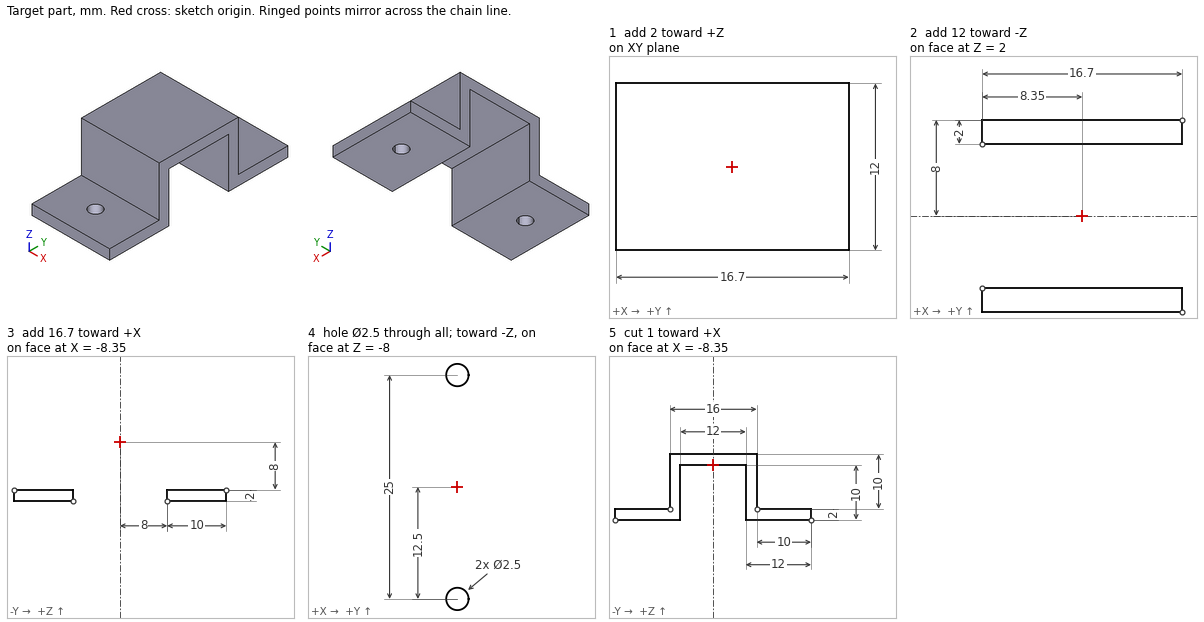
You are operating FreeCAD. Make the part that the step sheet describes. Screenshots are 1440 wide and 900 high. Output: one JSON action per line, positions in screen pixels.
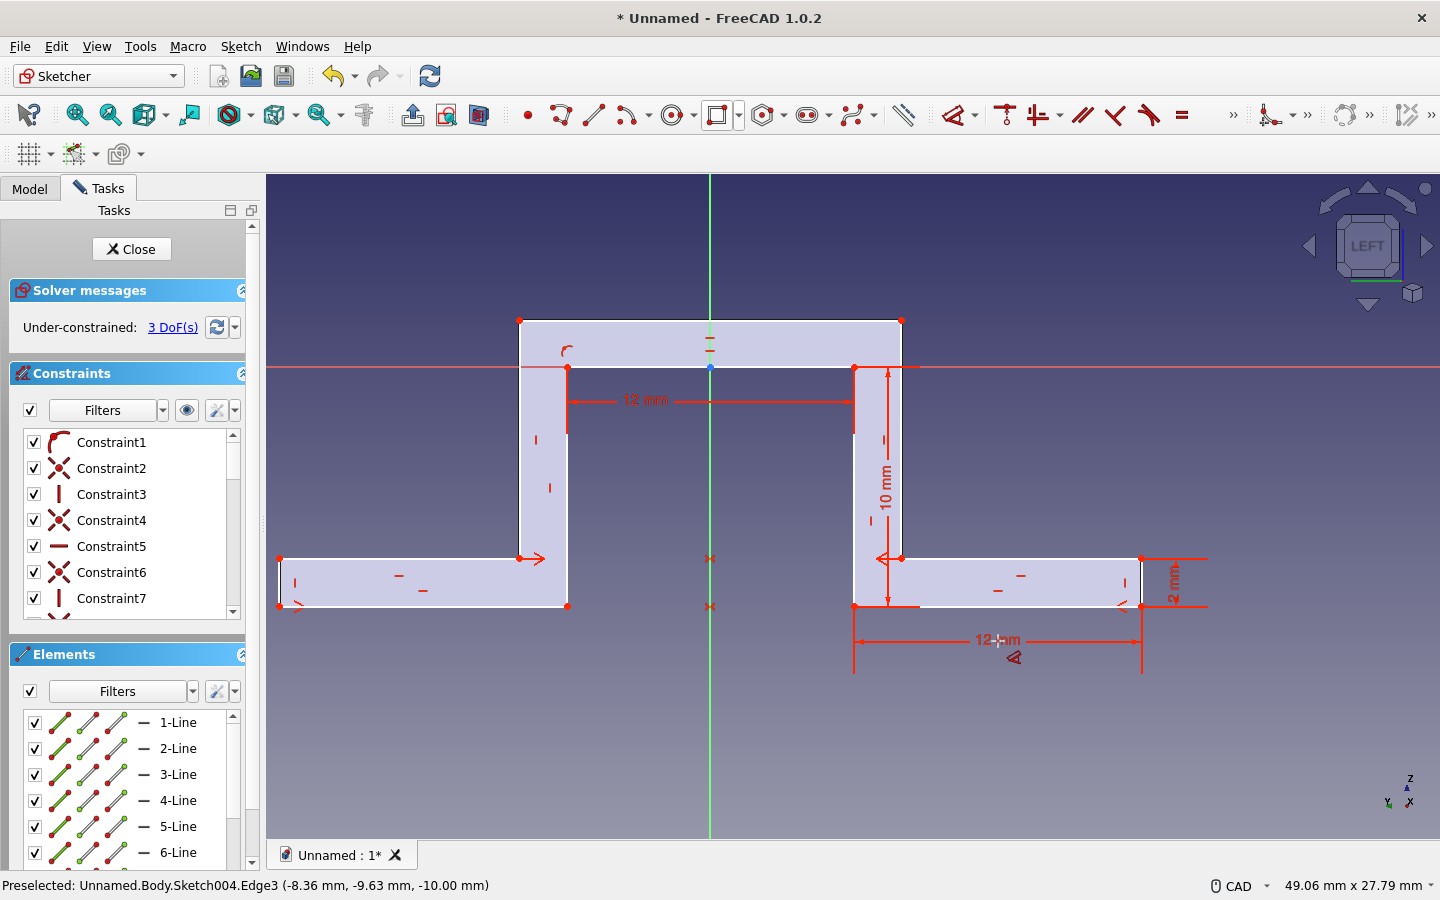
{"action": "left_click", "coordinate": [1070, 559]}
{"action": "left_click", "coordinate": [1022, 593]}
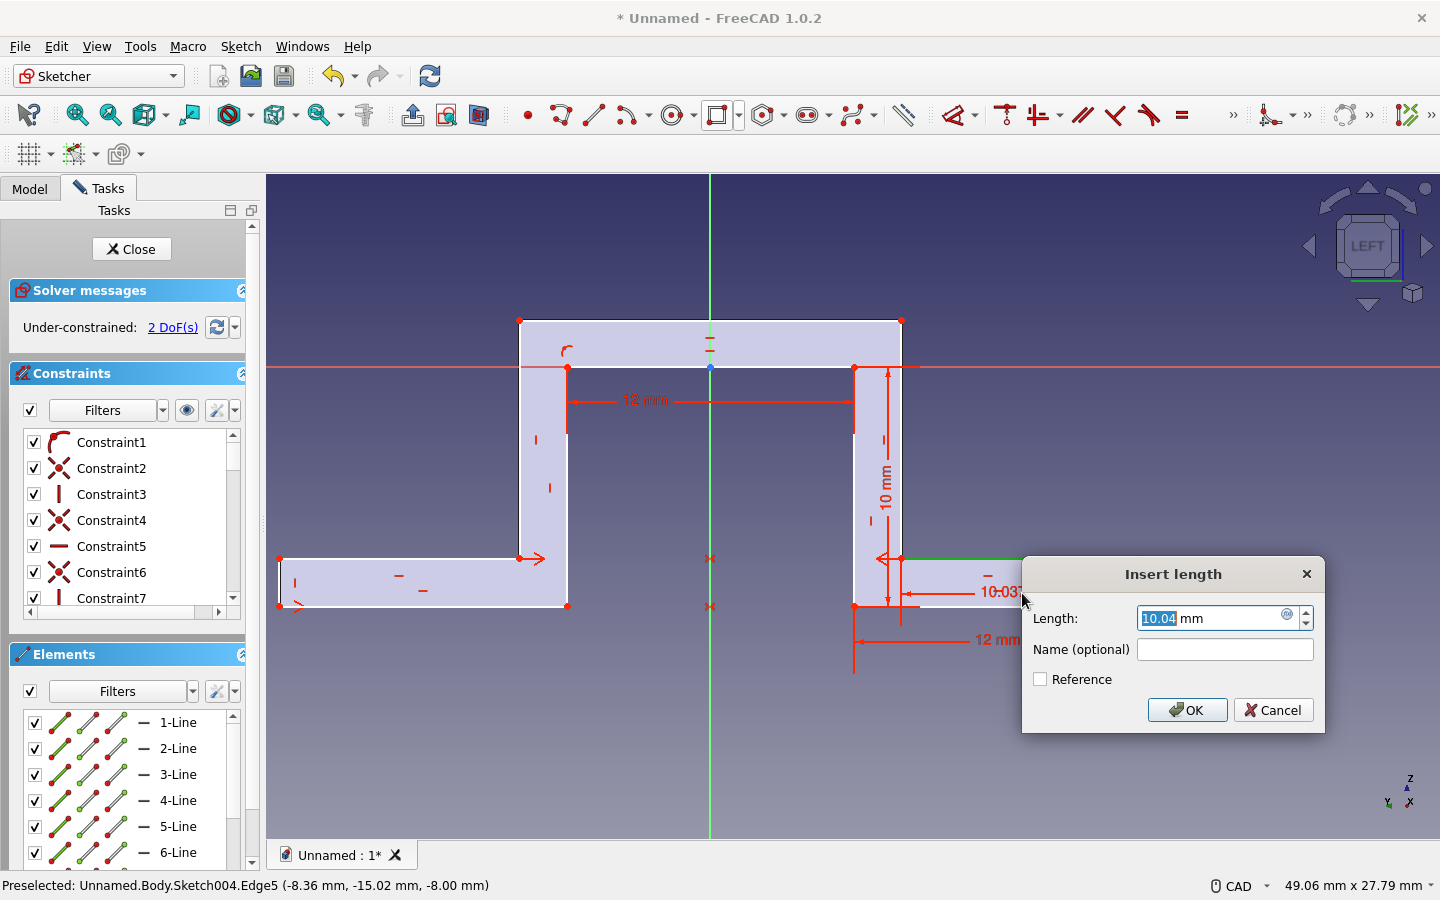
{"action": "type", "text": "10"}
{"action": "key", "text": "Return"}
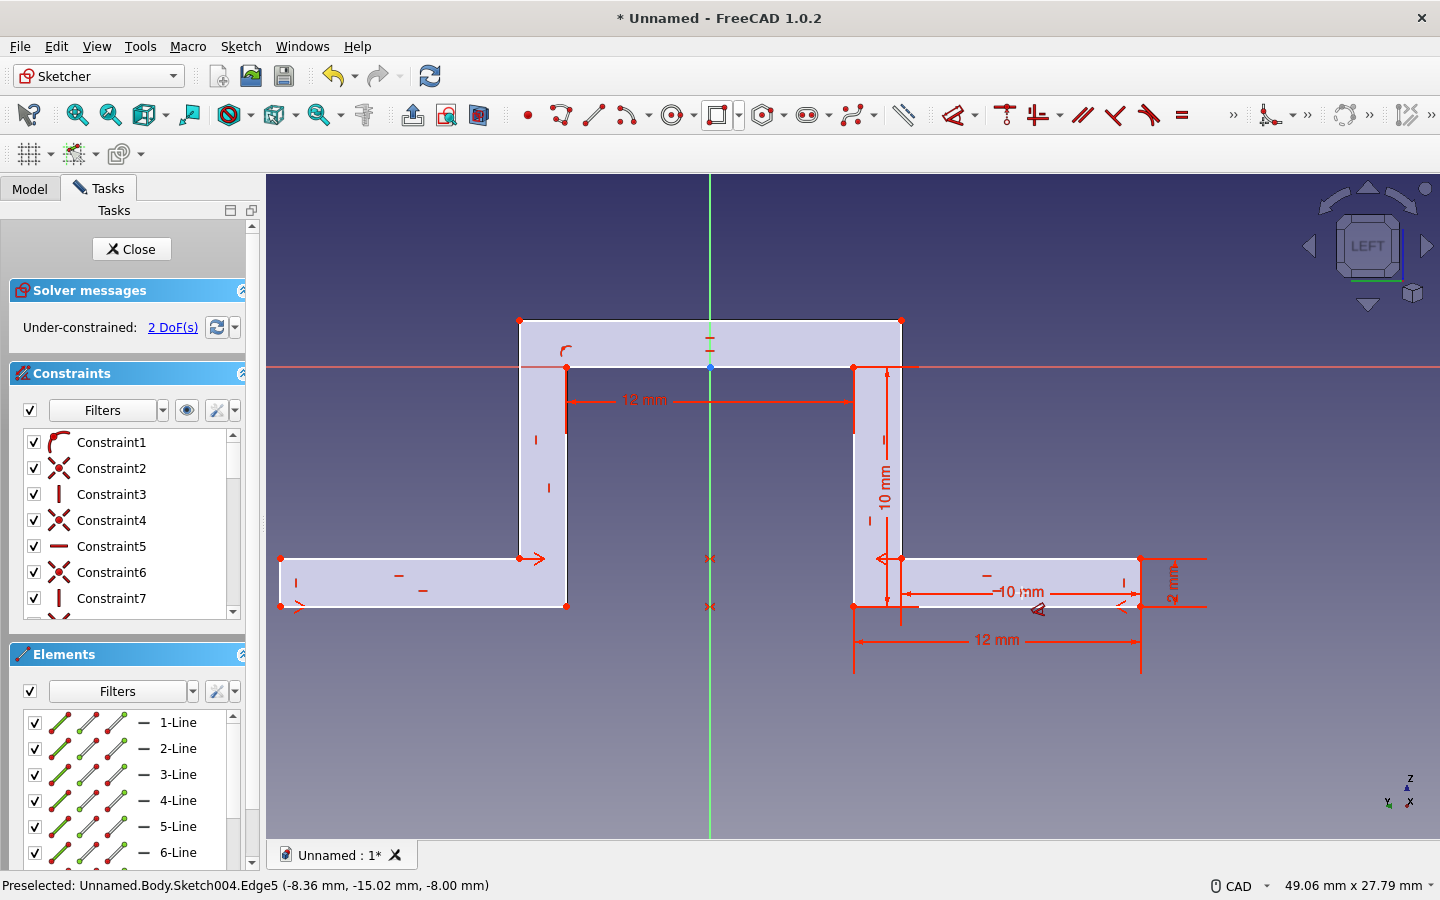
{"action": "left_click", "coordinate": [901, 487]}
{"action": "left_click", "coordinate": [935, 440]}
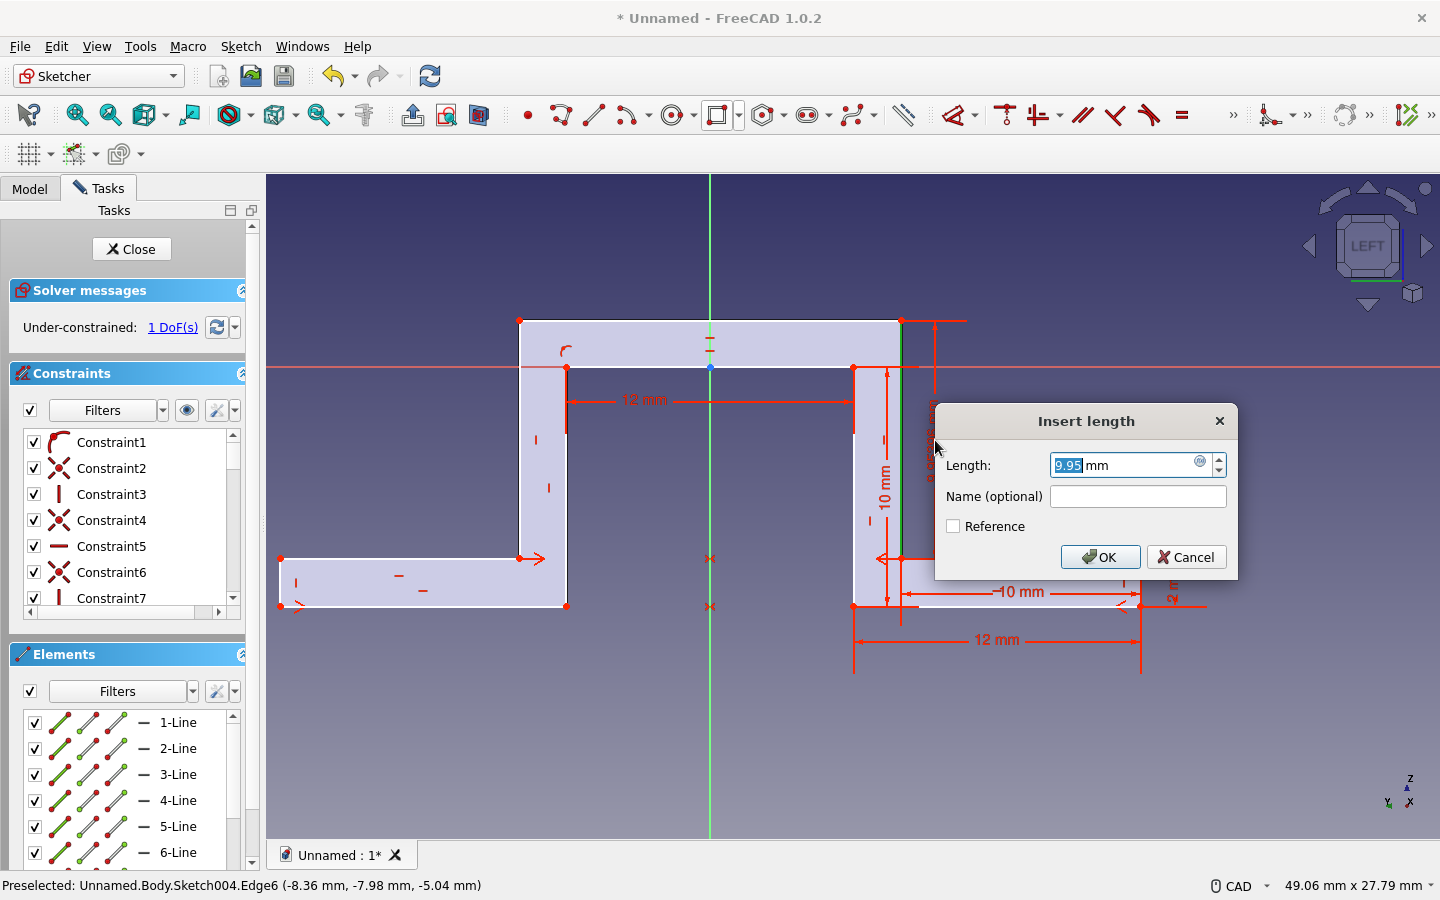
{"action": "type", "text": "10"}
{"action": "key", "text": "Return"}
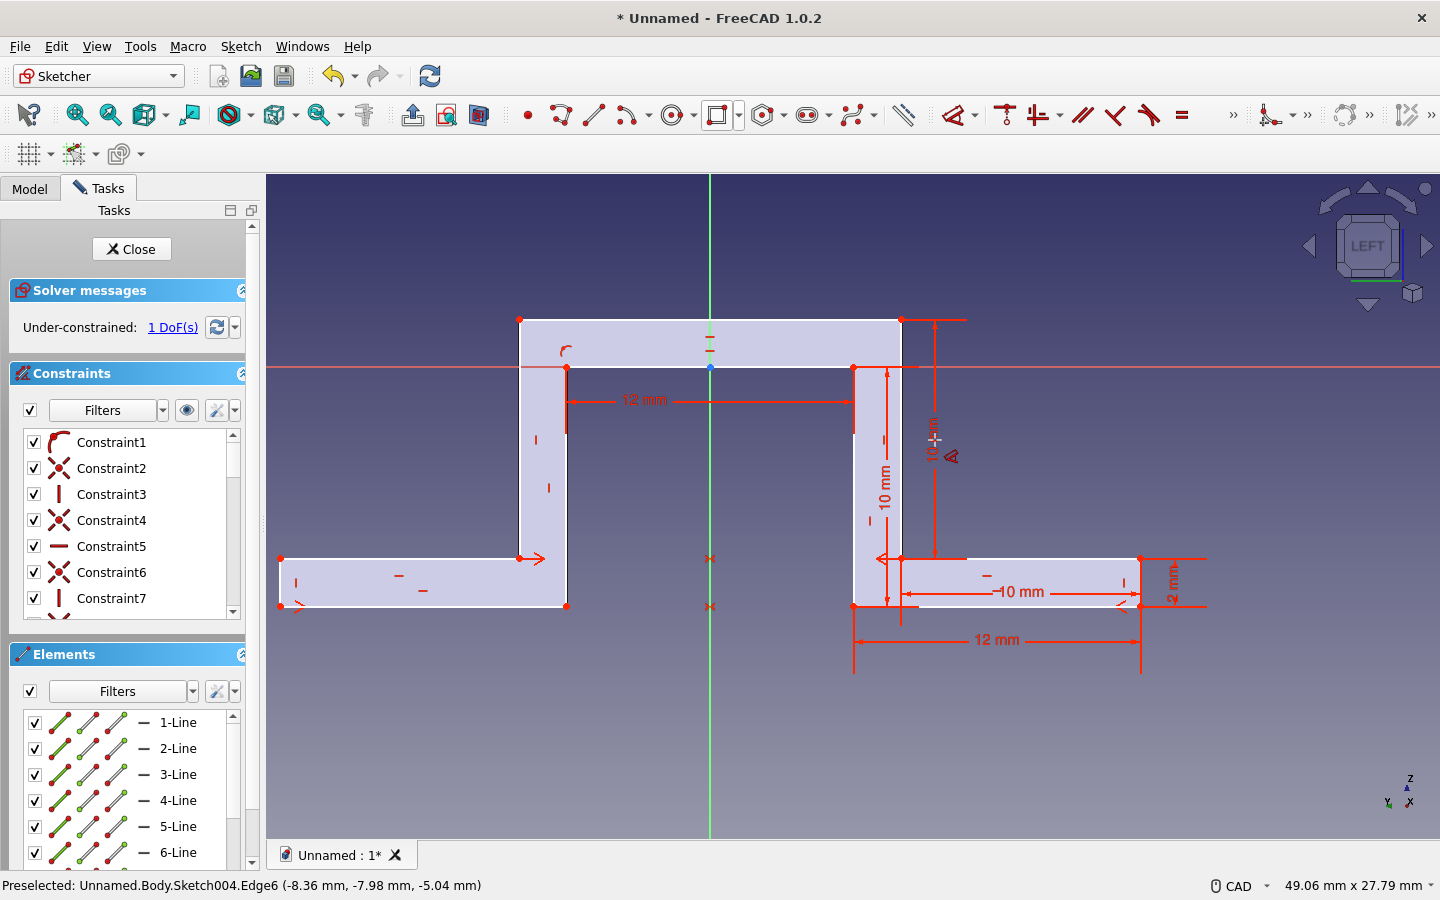
{"action": "left_click", "coordinate": [787, 320]}
{"action": "left_click", "coordinate": [623, 286]}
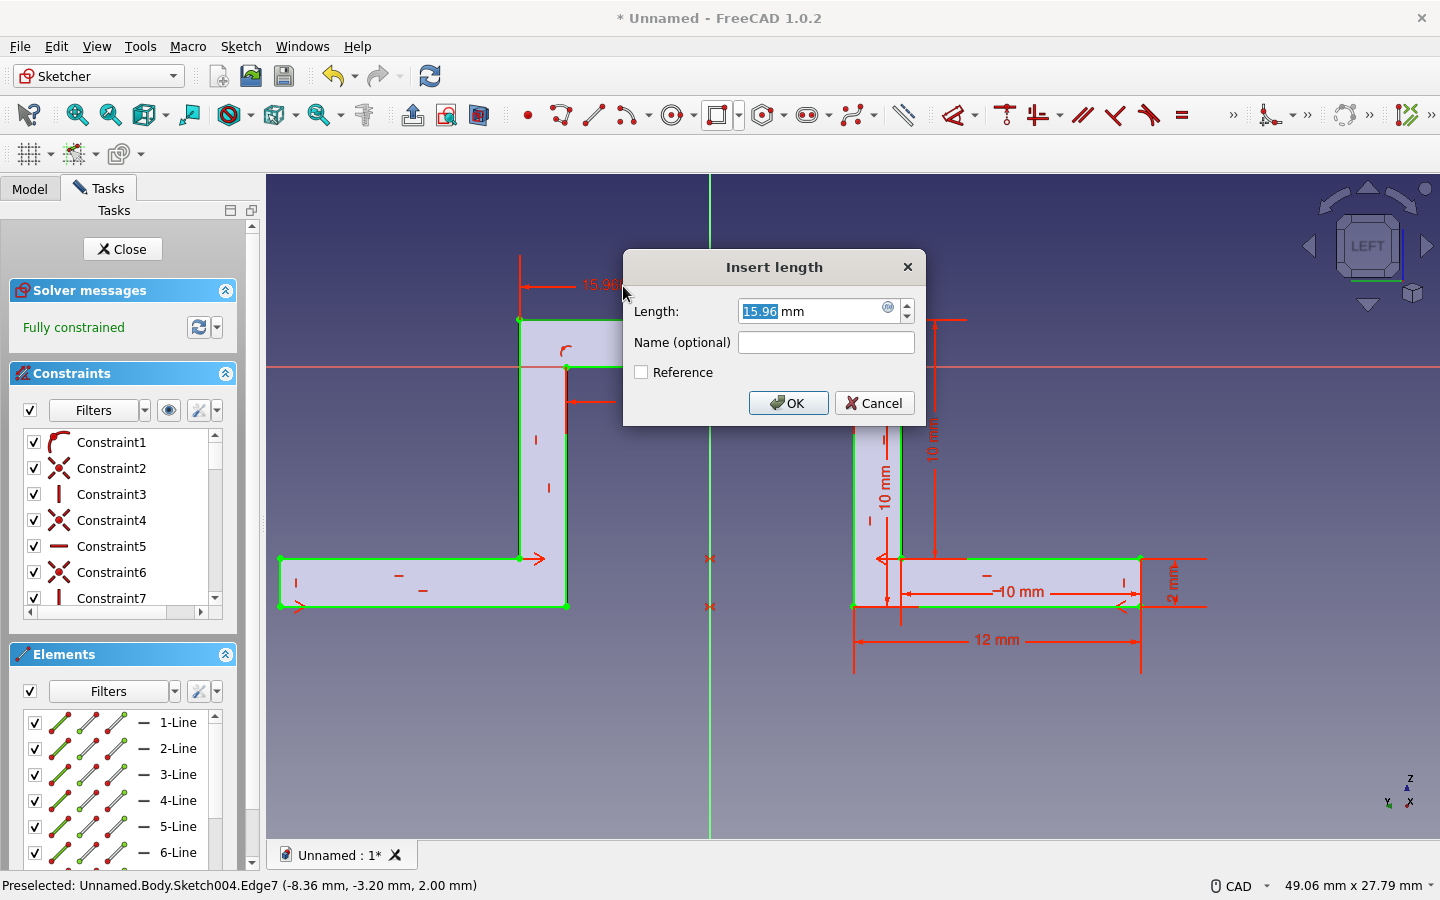
{"action": "type", "text": "16"}
{"action": "key", "text": "Return"}
{"action": "key", "text": "Escape"}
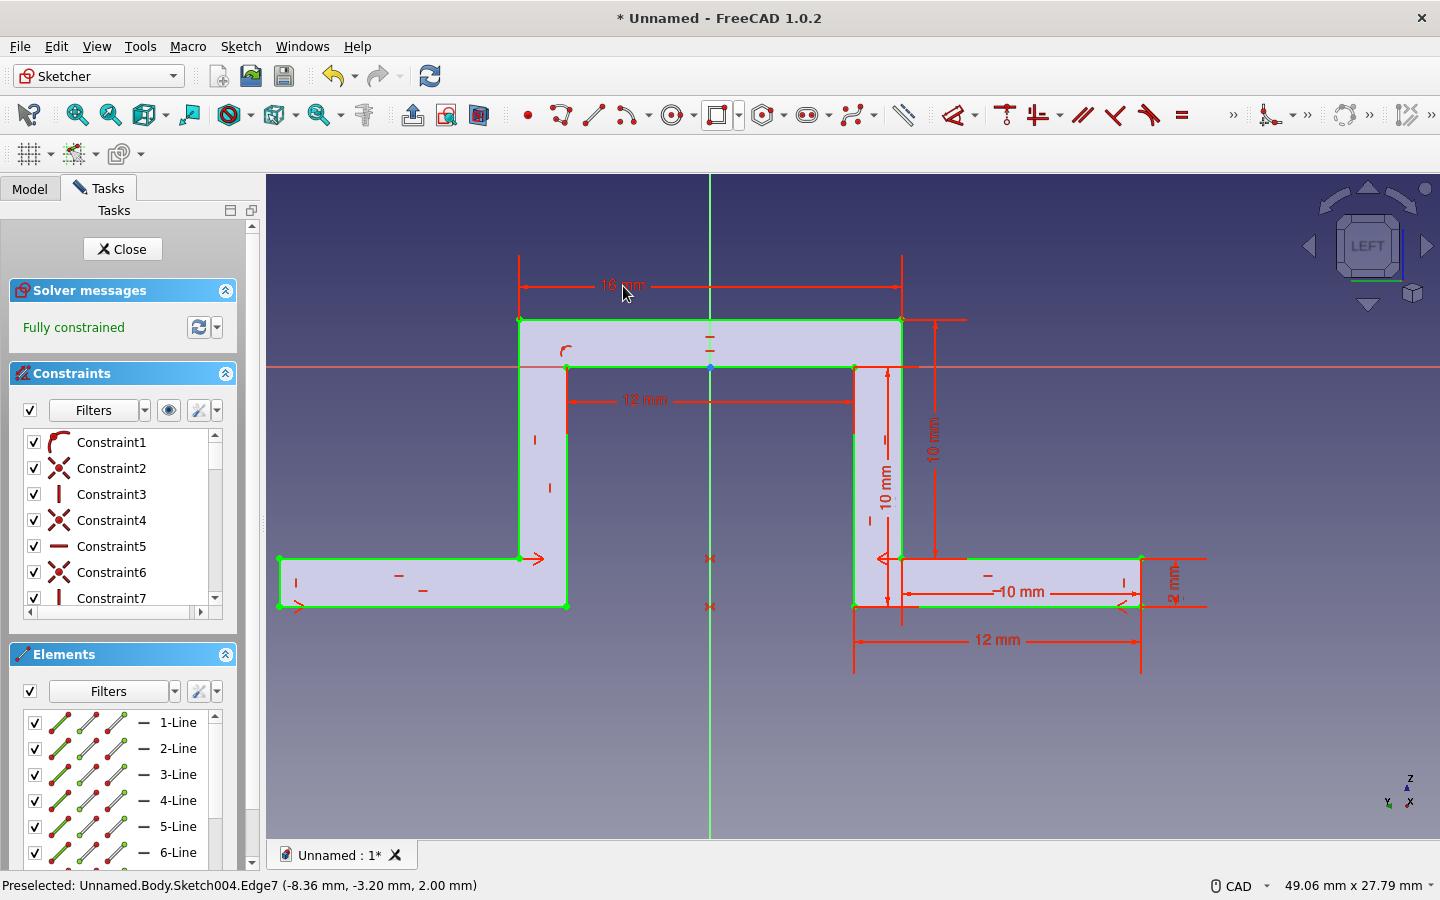
{"action": "left_click", "coordinate": [123, 249]}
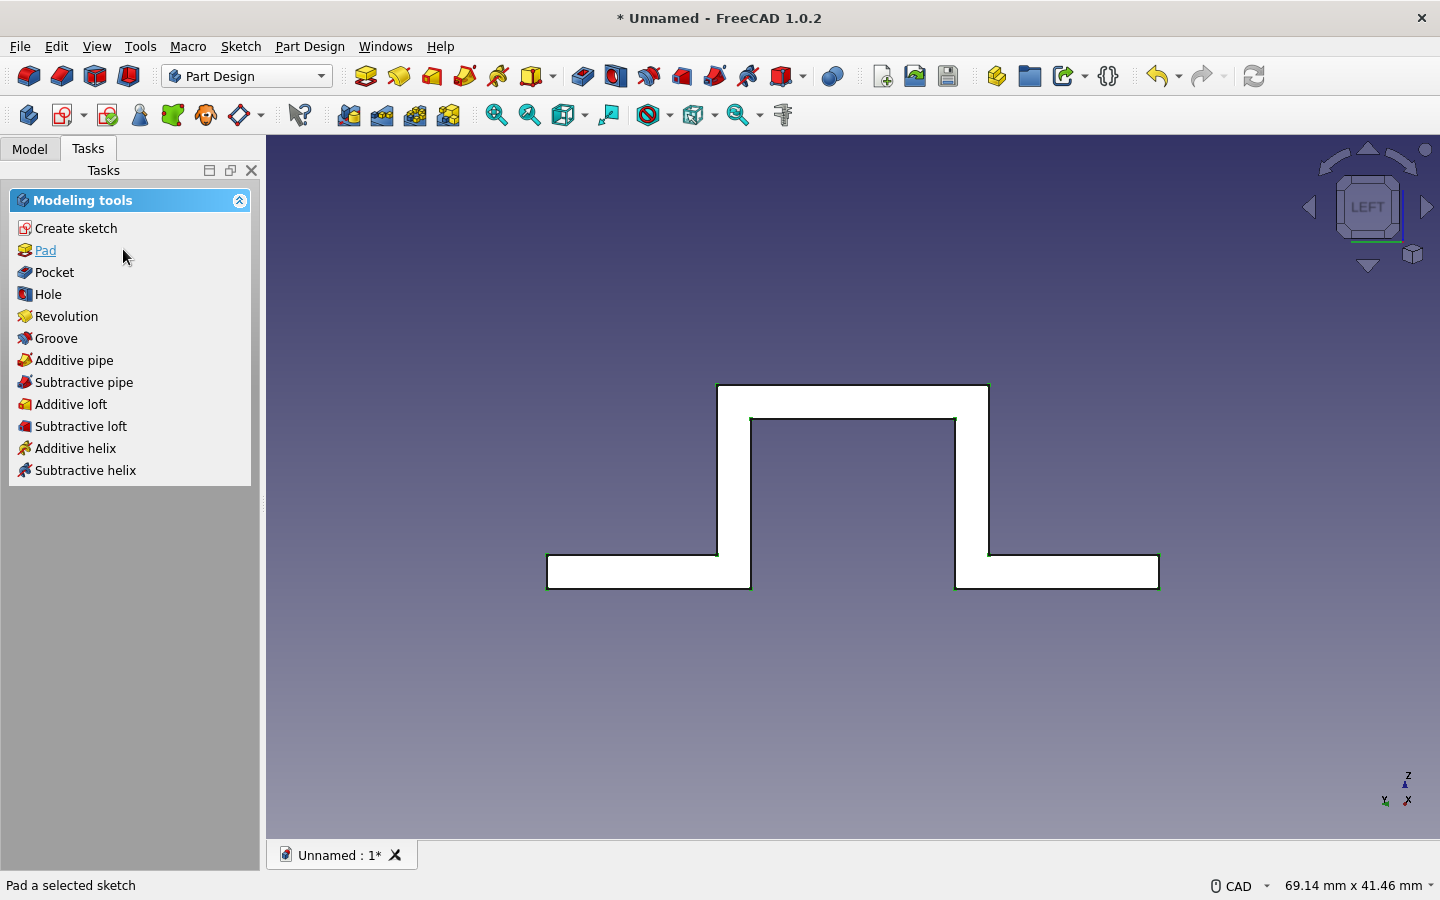
{"action": "left_click", "coordinate": [583, 76]}